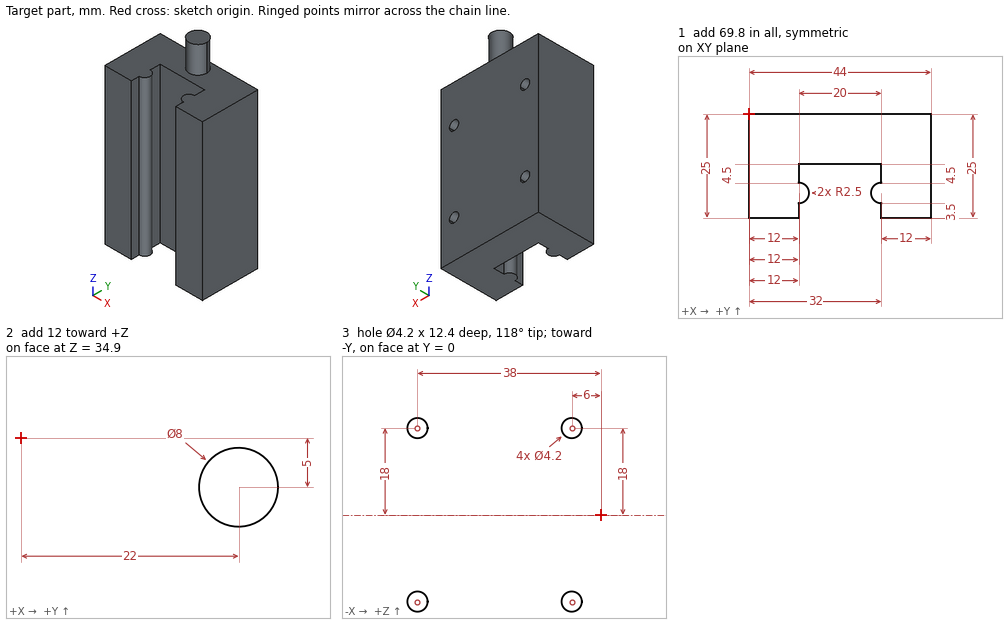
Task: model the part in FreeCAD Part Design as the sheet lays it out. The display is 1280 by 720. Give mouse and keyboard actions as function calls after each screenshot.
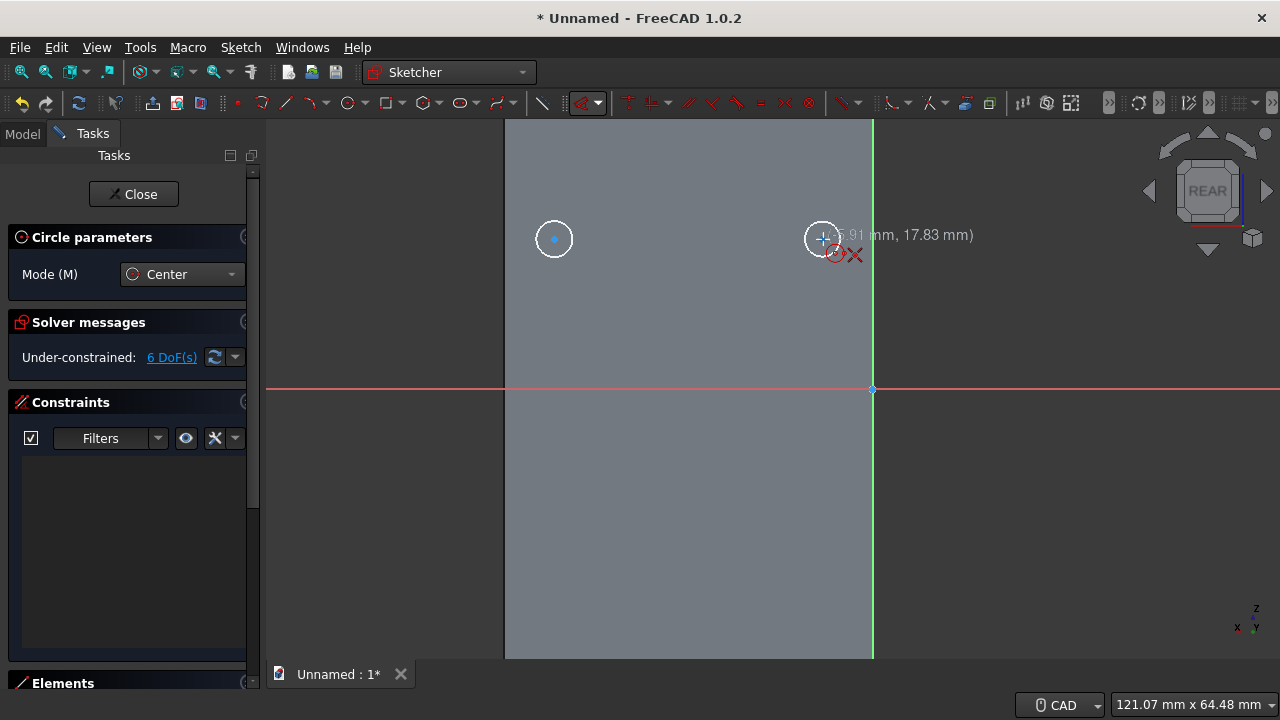
scroll(822, 540, up, 2)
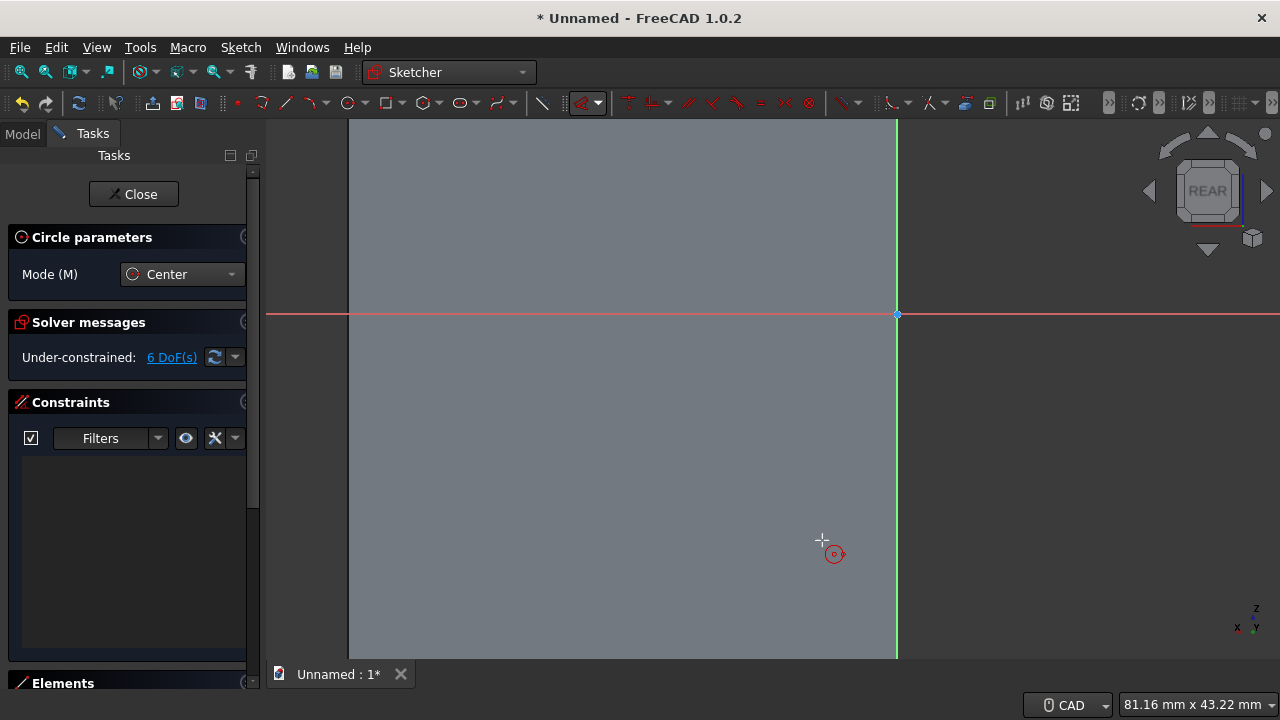
click(822, 539)
click(841, 521)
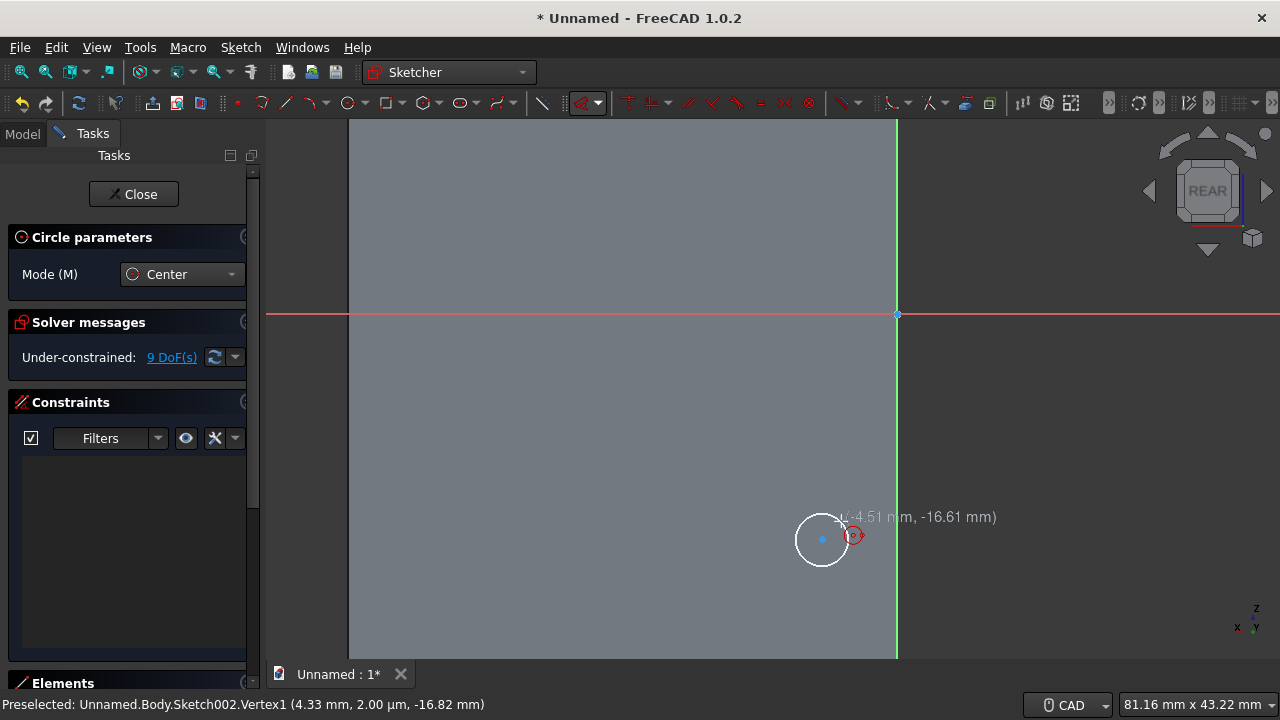
click(423, 539)
click(441, 521)
key(Escape)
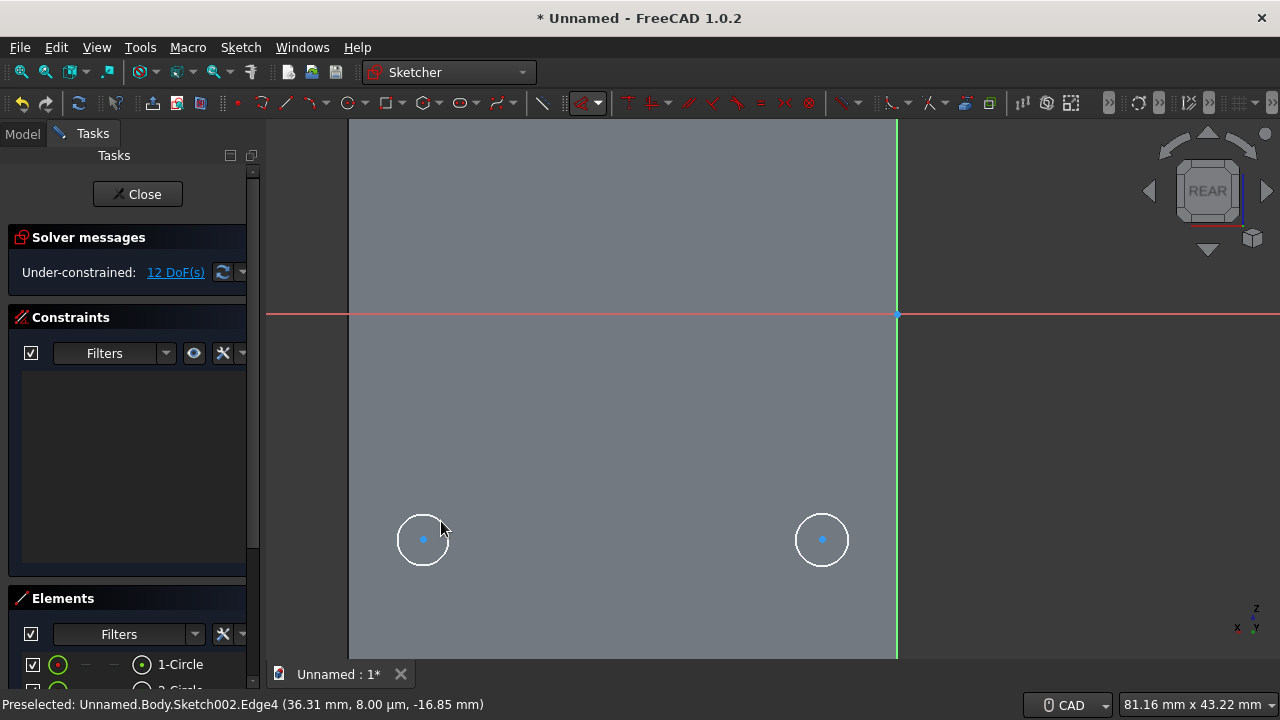
scroll(822, 541, down, 2)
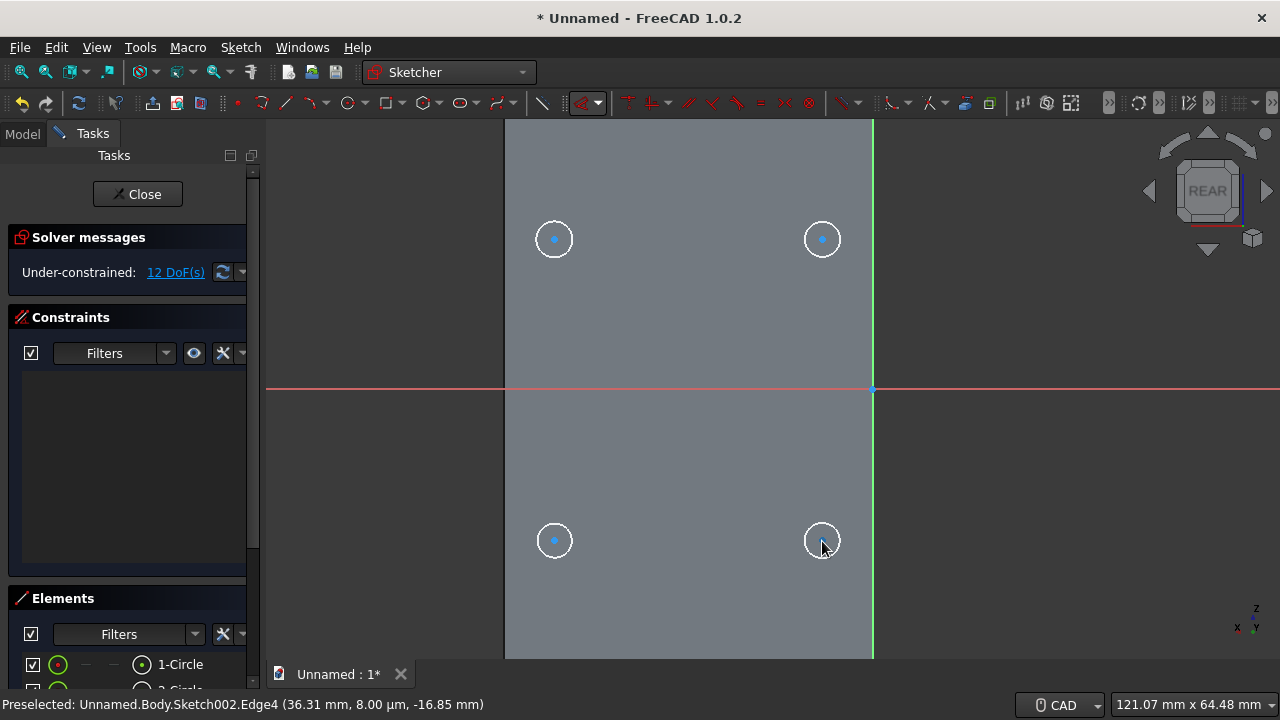
click(835, 227)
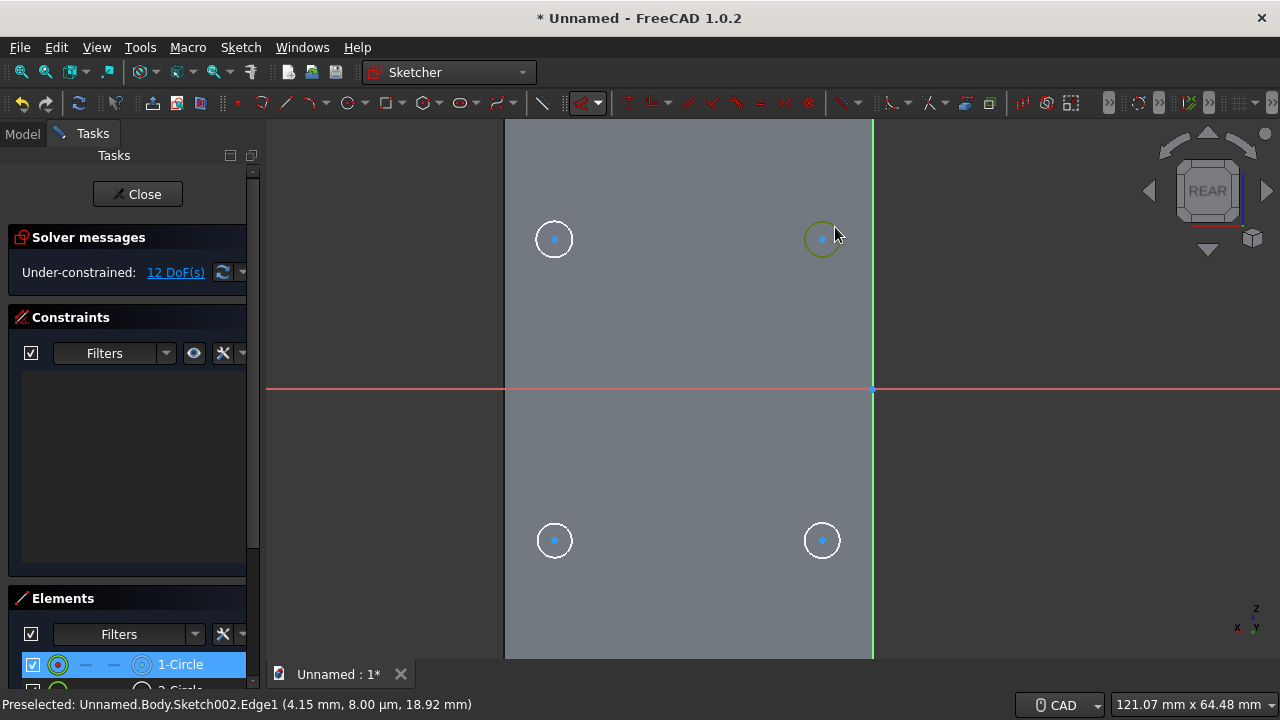
click(567, 227)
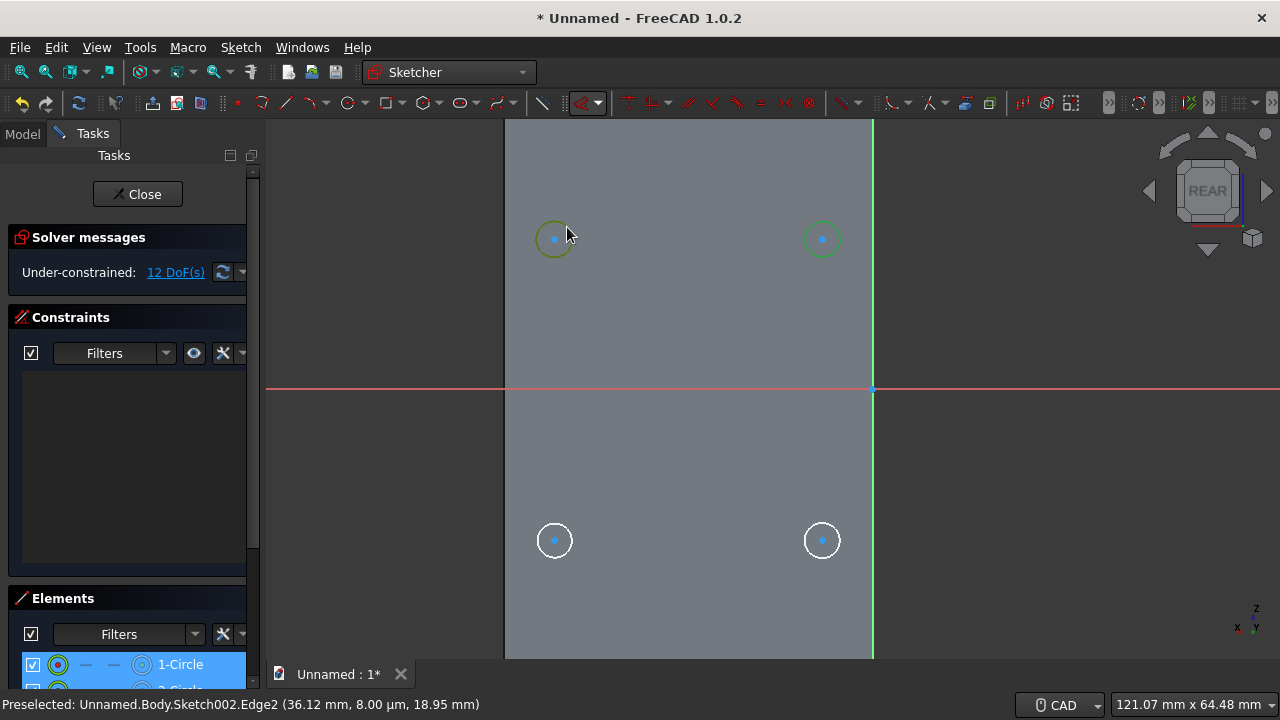
click(835, 528)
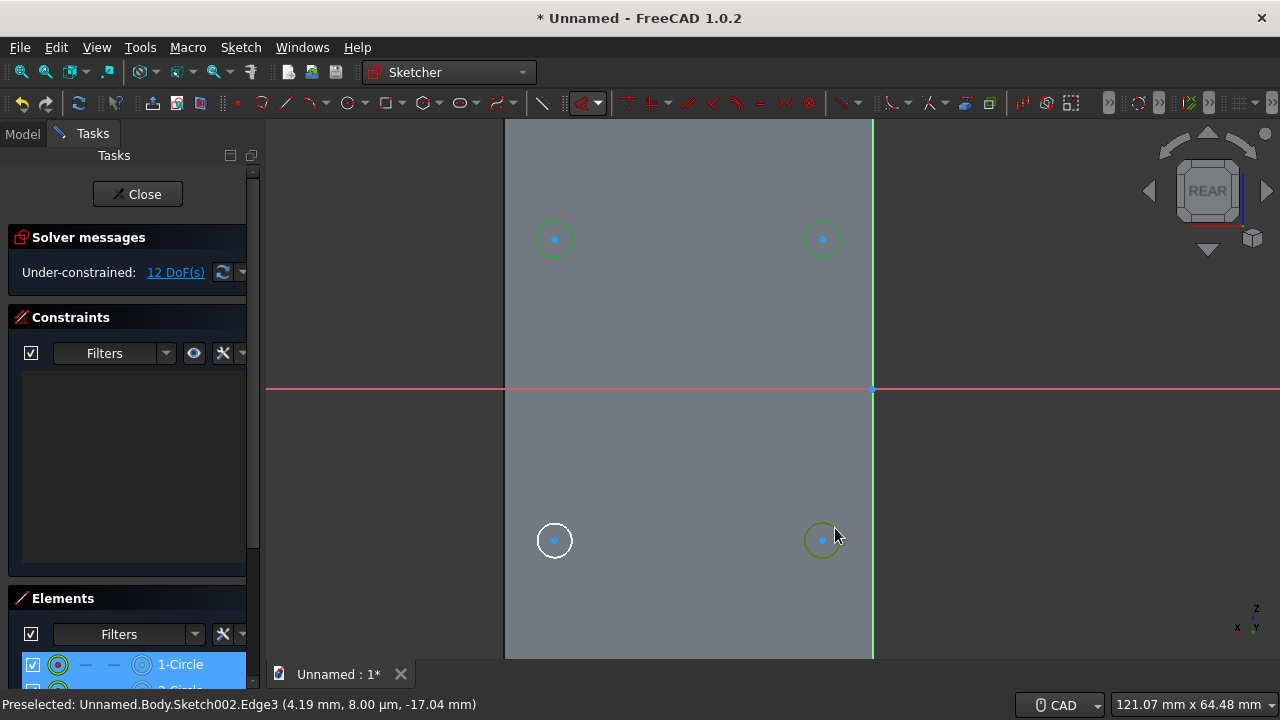
click(567, 528)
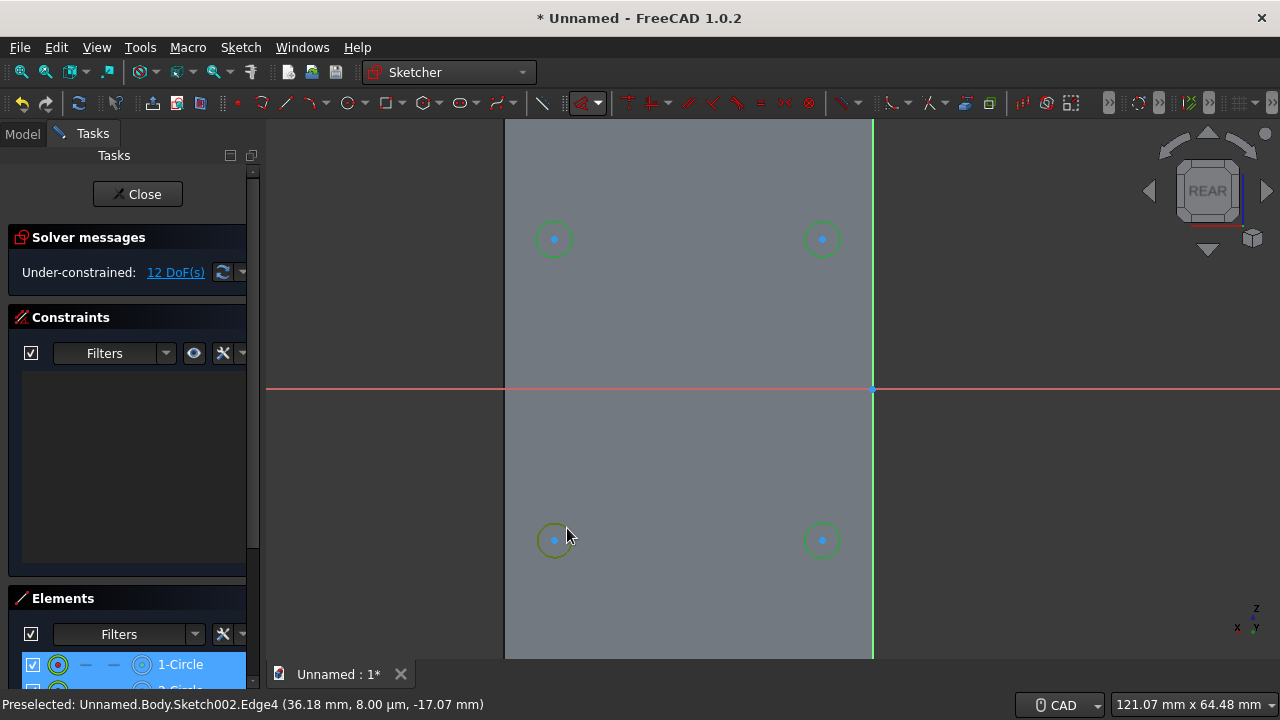
click(762, 104)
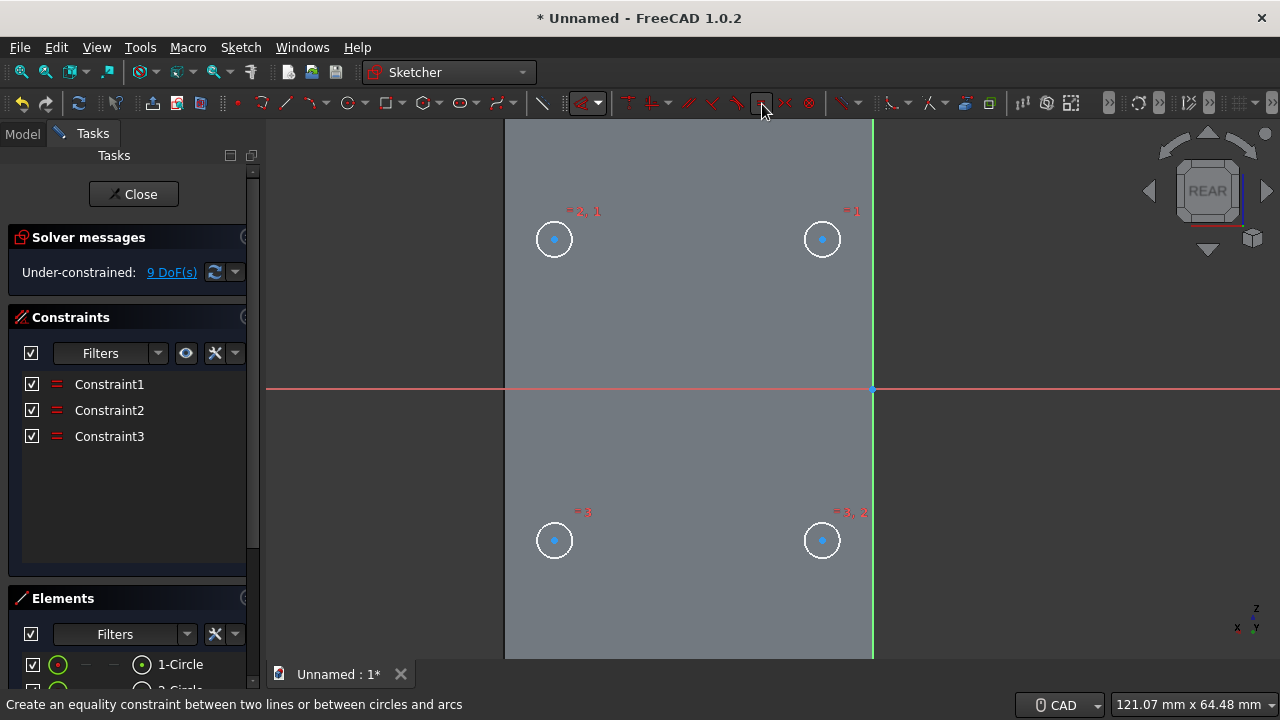
click(823, 239)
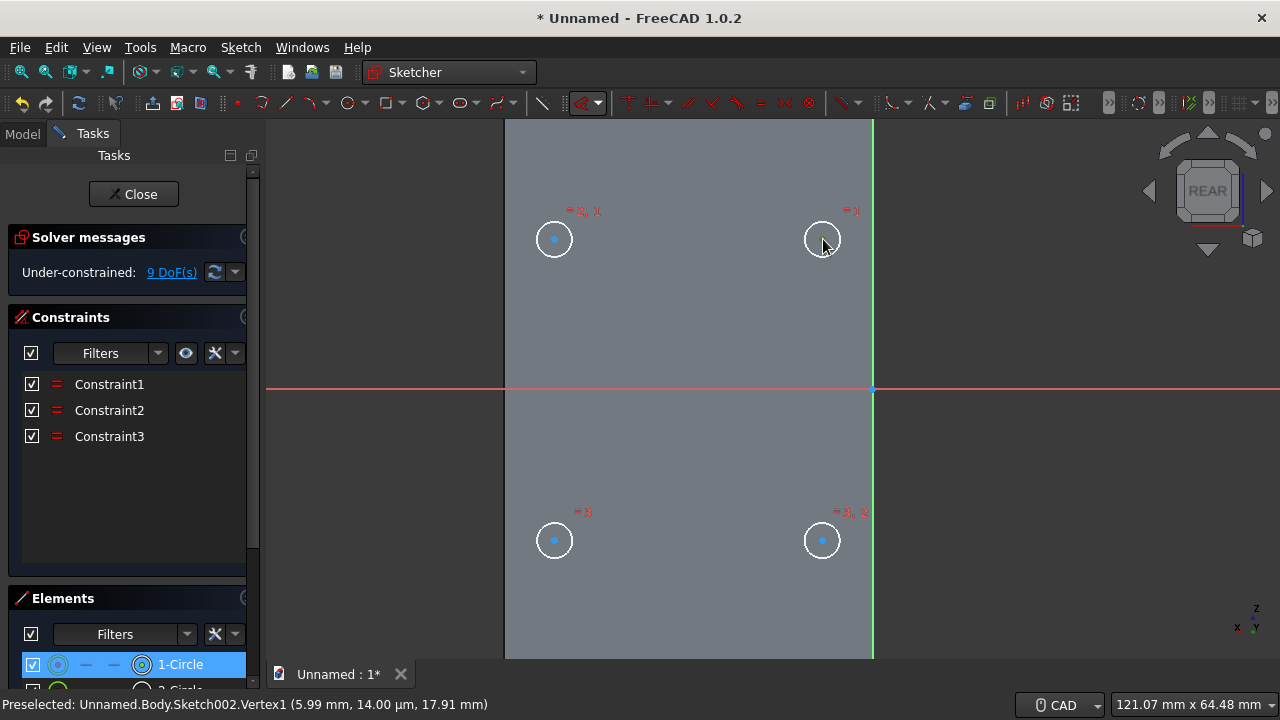
click(822, 541)